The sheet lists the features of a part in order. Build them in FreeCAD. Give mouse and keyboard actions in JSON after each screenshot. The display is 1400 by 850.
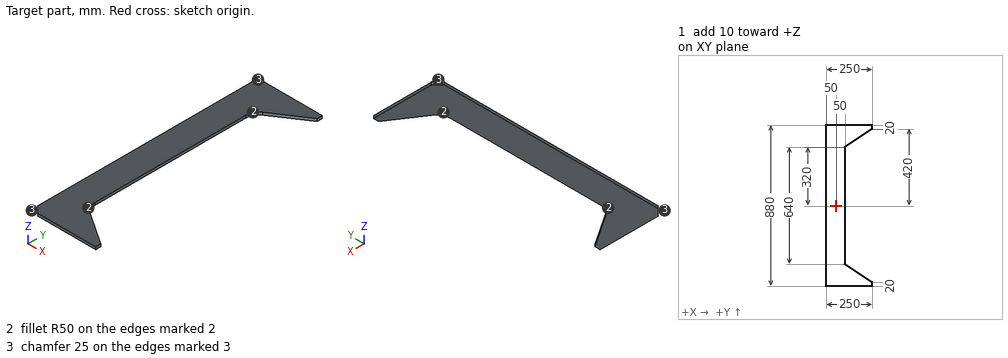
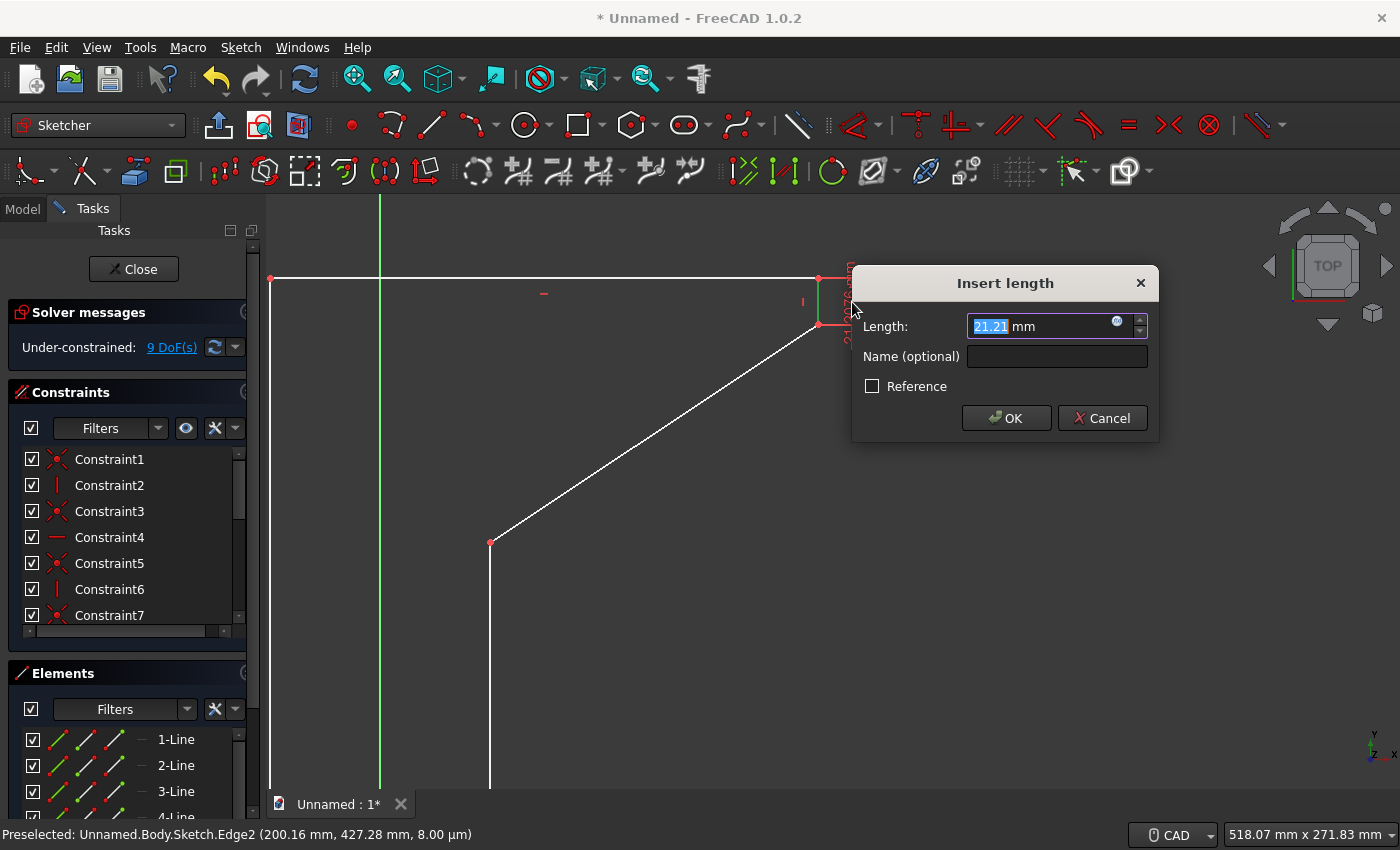
{"action": "type", "text": "20"}
{"action": "key", "text": "Return"}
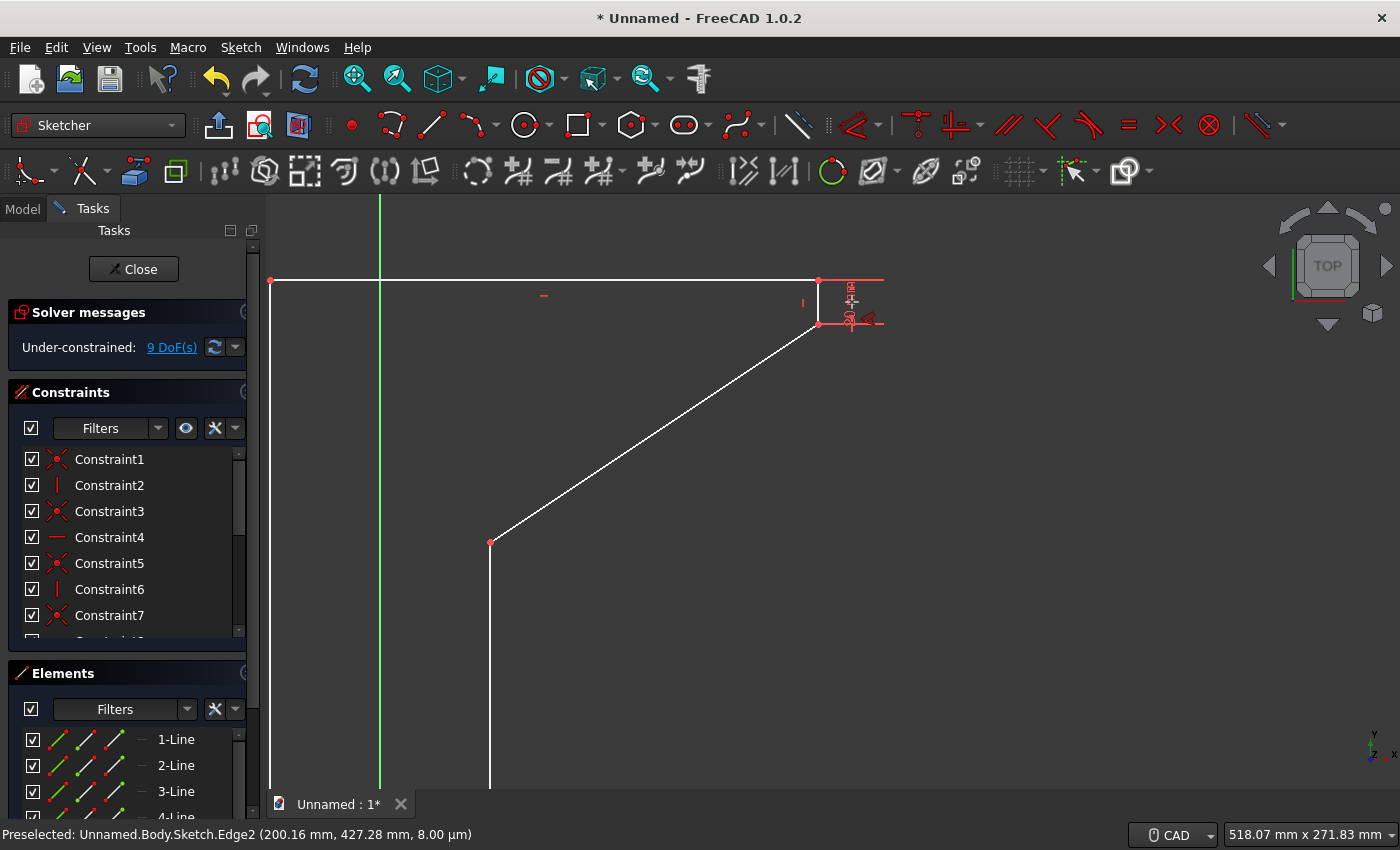
{"action": "scroll", "coordinate": [820, 303], "scroll_direction": "down", "scroll_amount": 8}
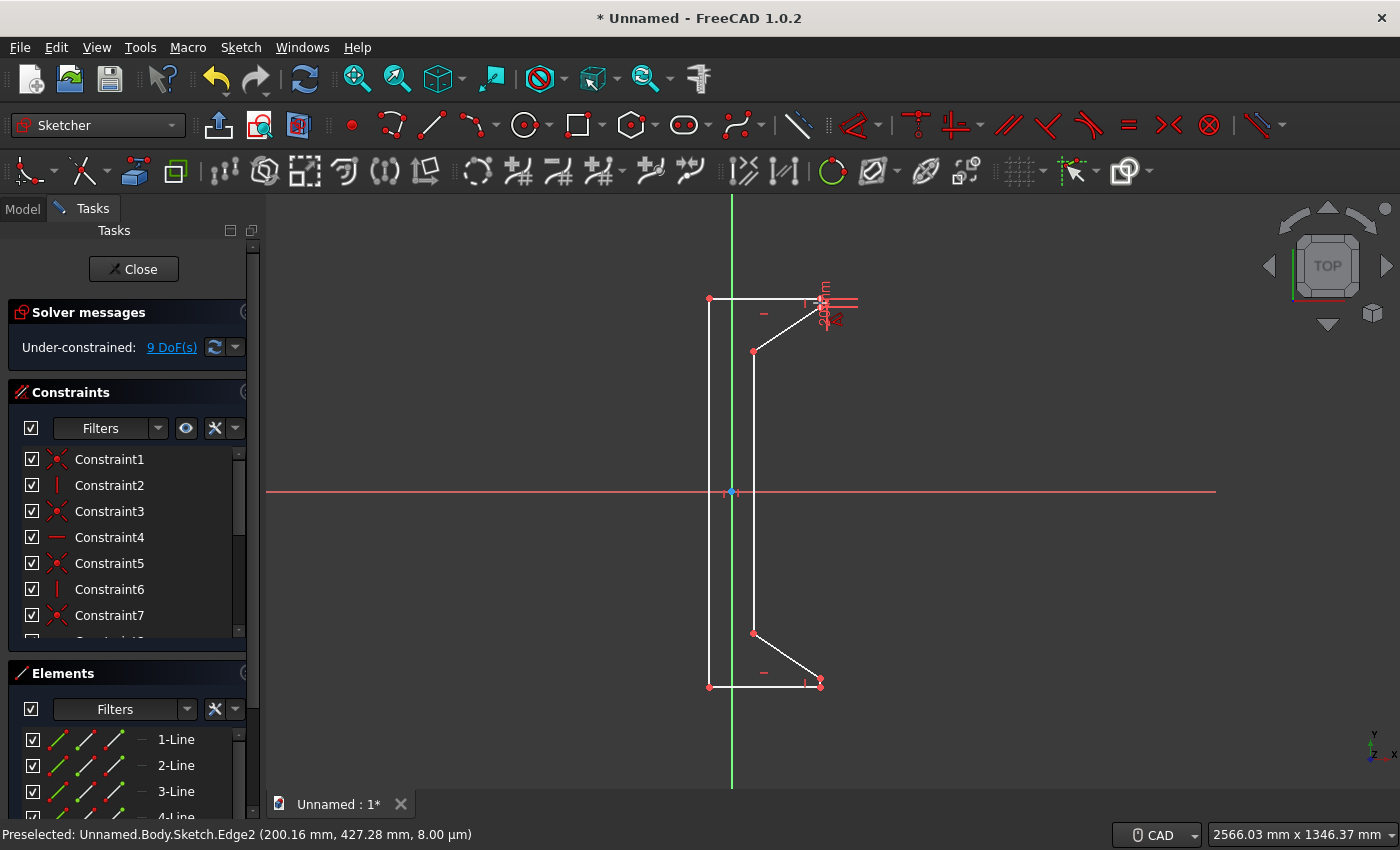
{"action": "scroll", "coordinate": [820, 685], "scroll_direction": "up", "scroll_amount": 9}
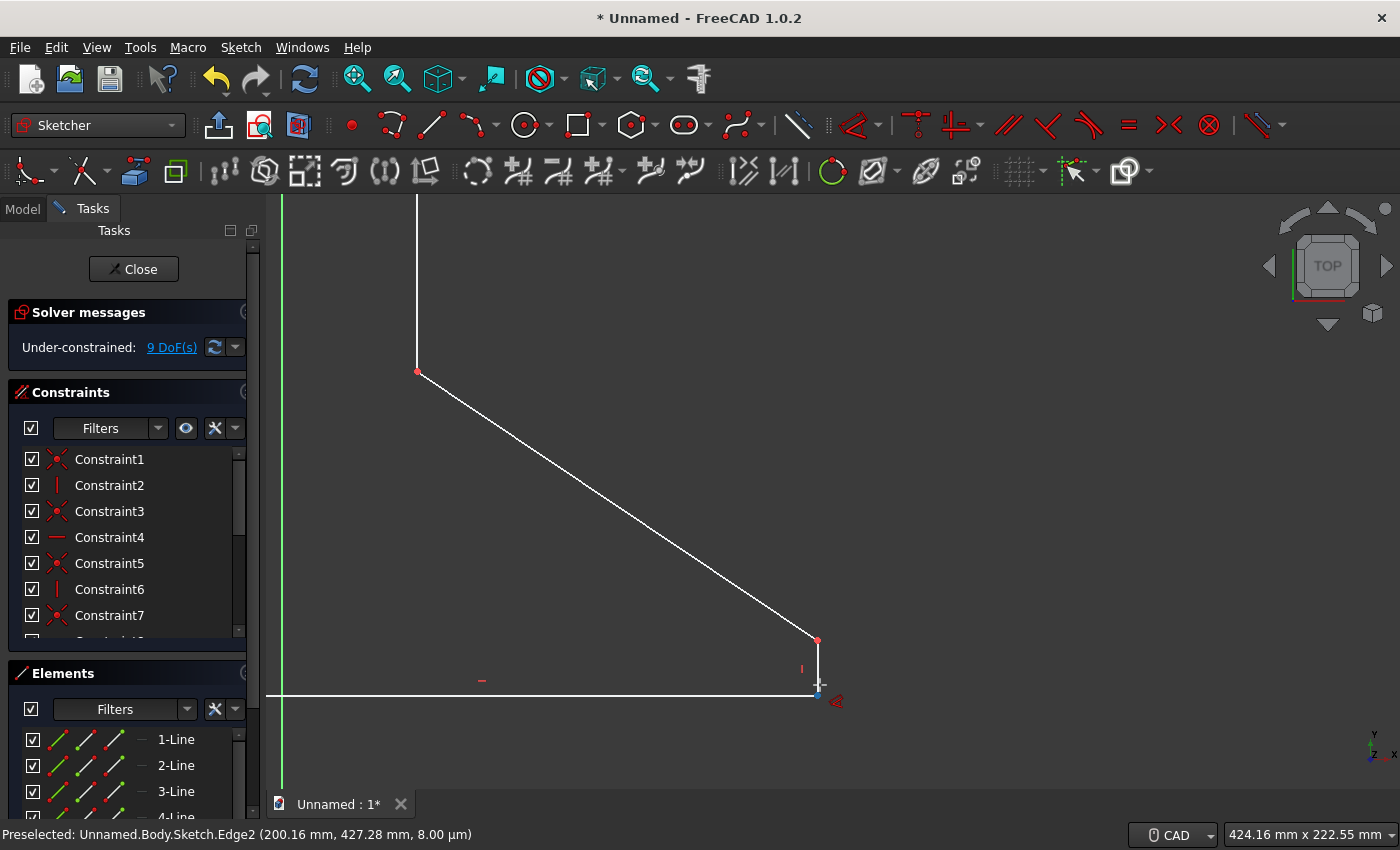
{"action": "left_click", "coordinate": [818, 679]}
{"action": "left_click", "coordinate": [852, 668]}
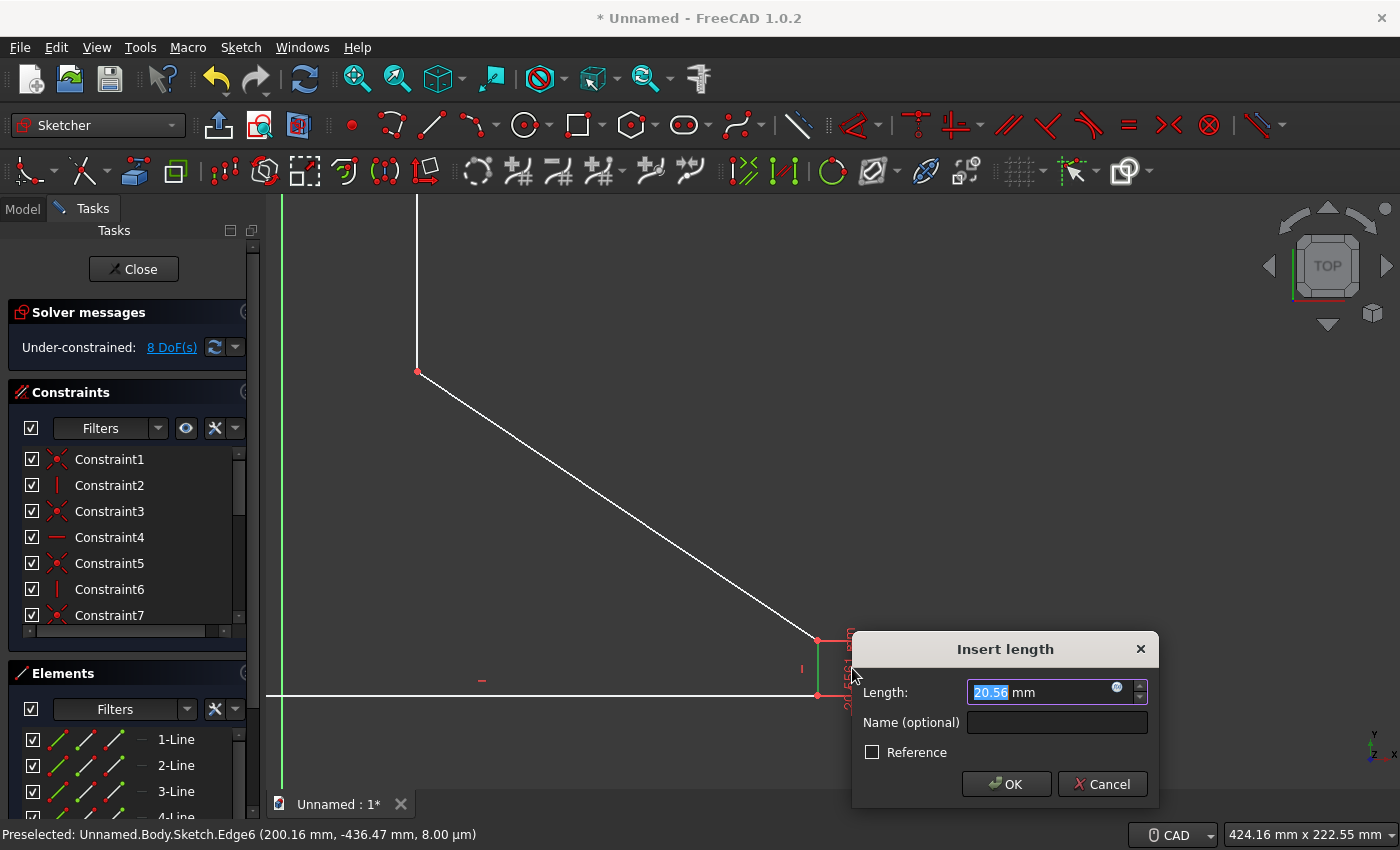
{"action": "type", "text": "20"}
{"action": "key", "text": "Return"}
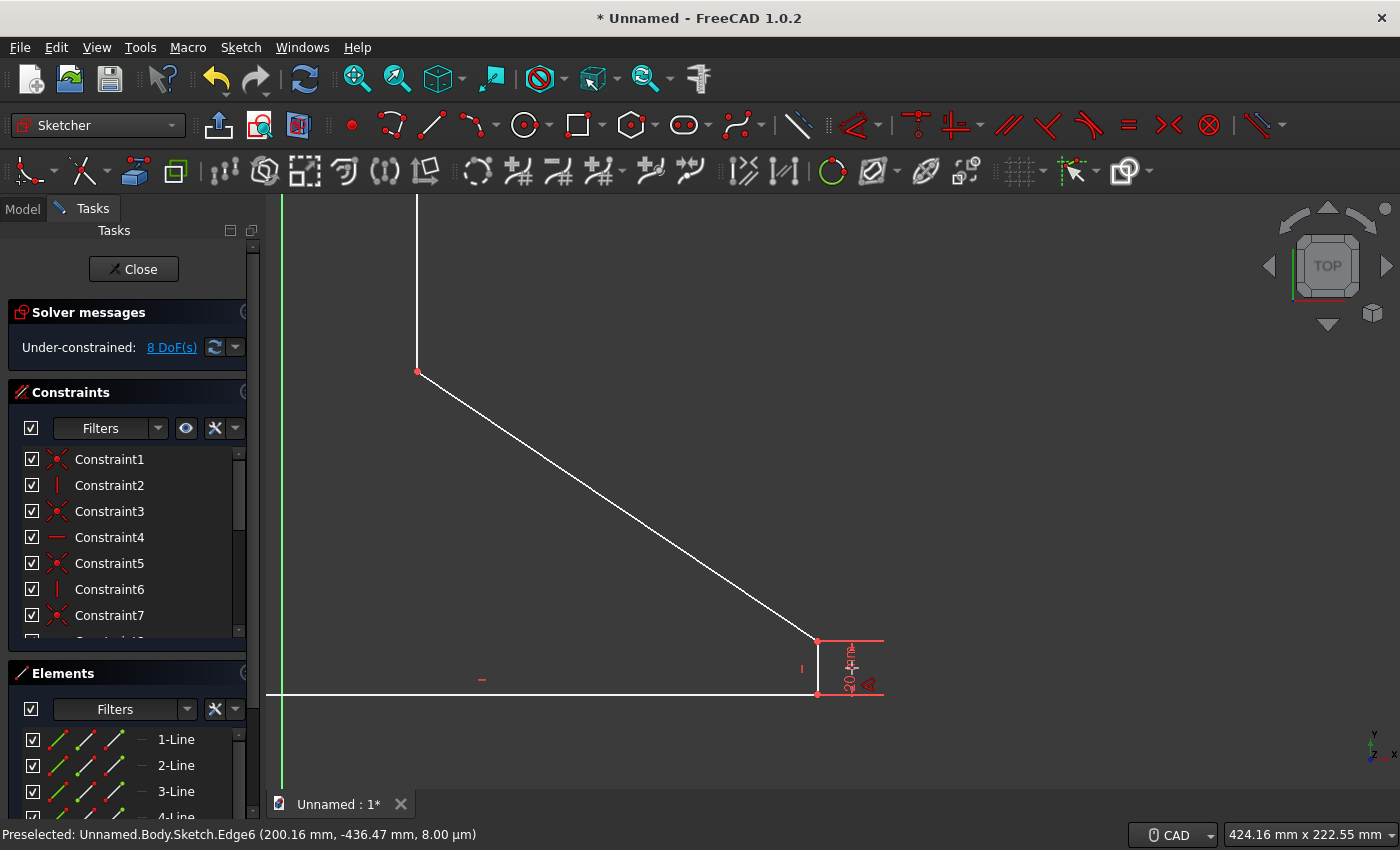
{"action": "scroll", "coordinate": [820, 685], "scroll_direction": "down", "scroll_amount": 9}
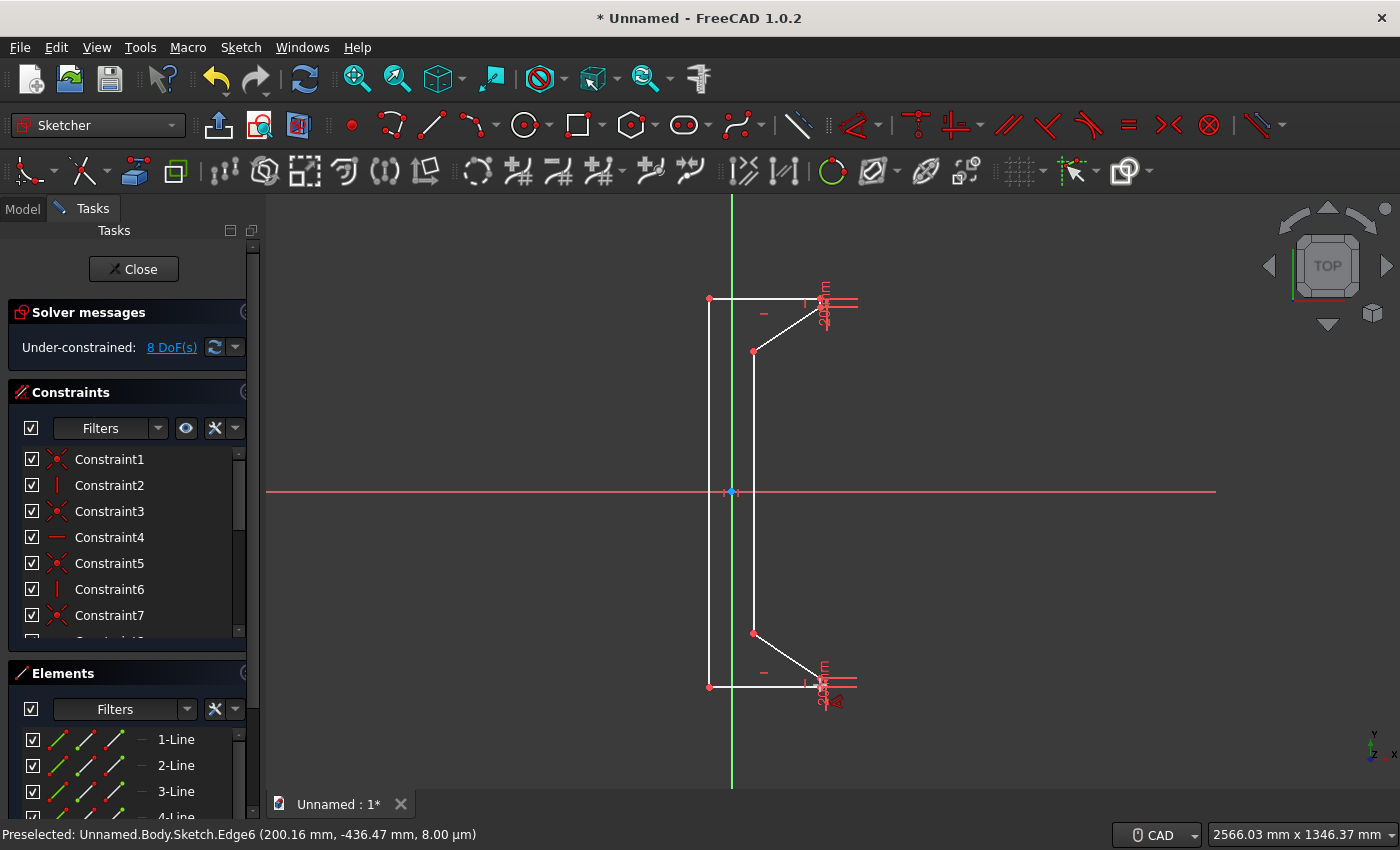
{"action": "left_click", "coordinate": [787, 299]}
{"action": "left_click", "coordinate": [765, 265]}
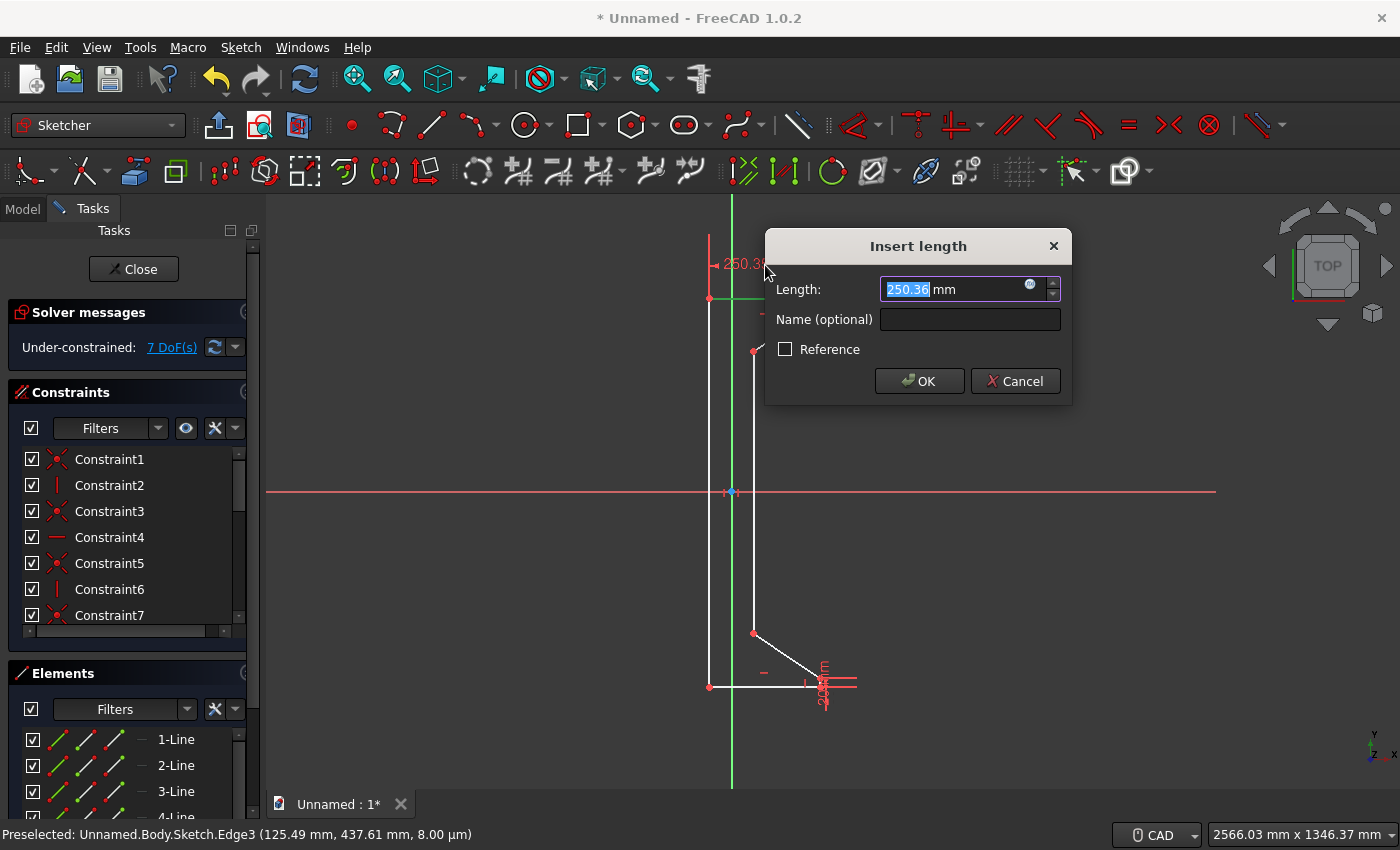
{"action": "type", "text": "250"}
{"action": "key", "text": "Return"}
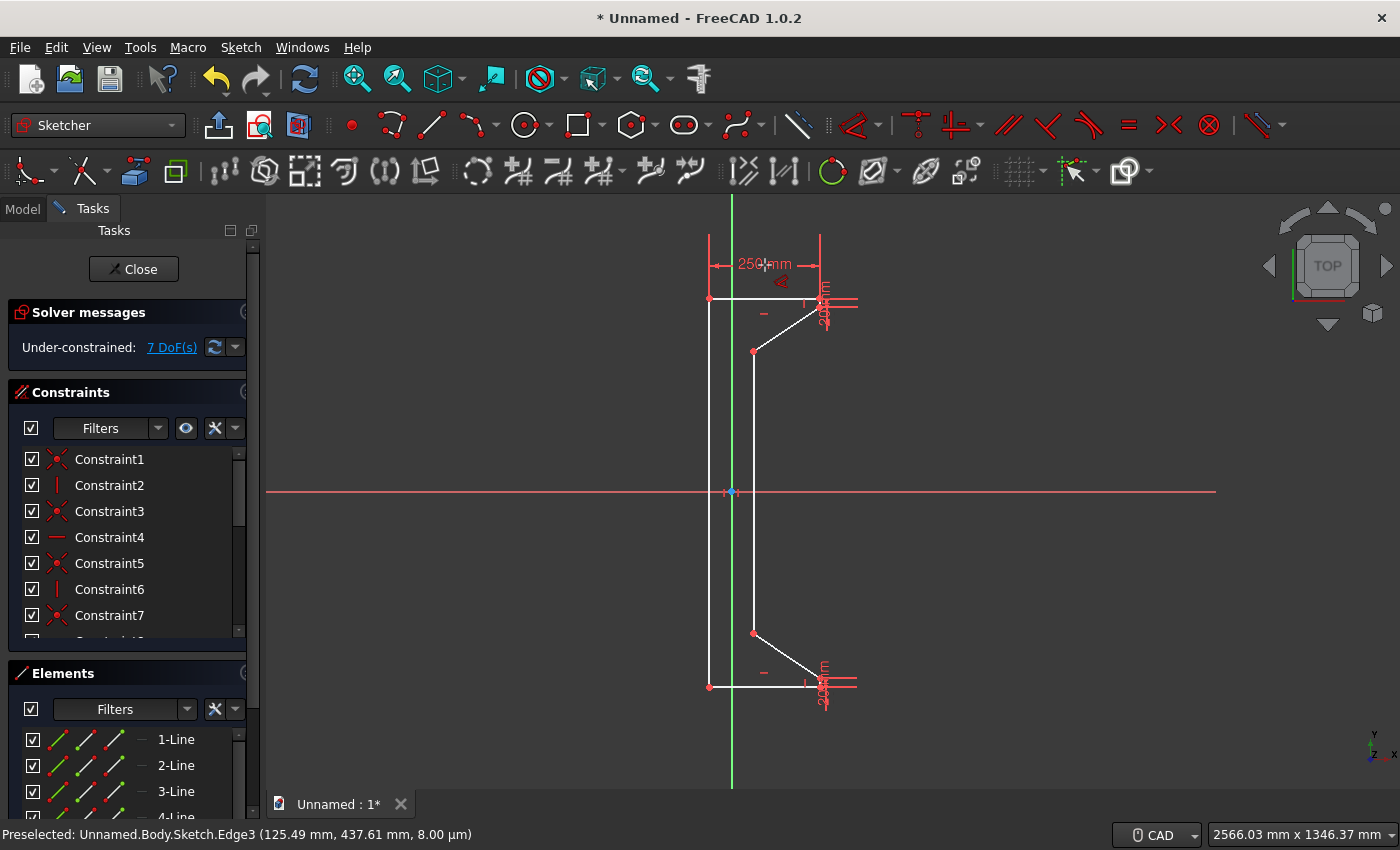
{"action": "left_click", "coordinate": [709, 415]}
{"action": "left_click", "coordinate": [675, 404]}